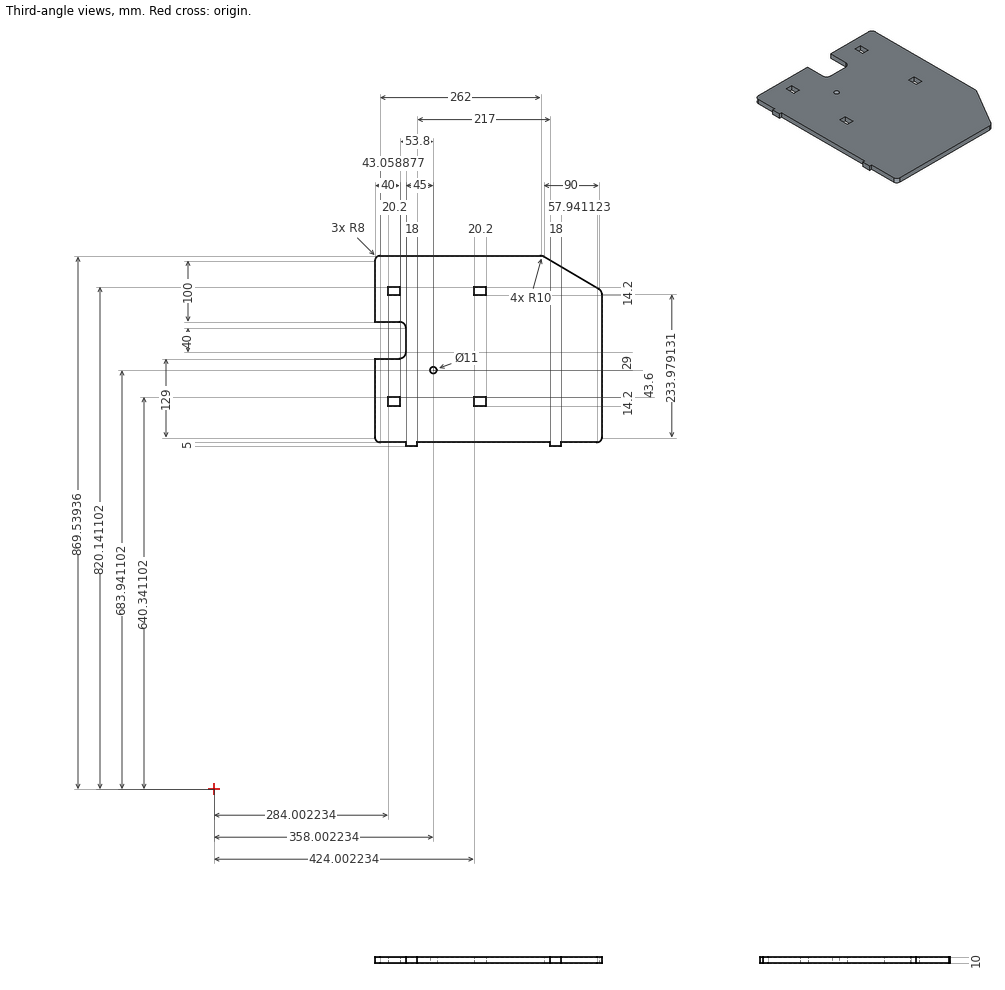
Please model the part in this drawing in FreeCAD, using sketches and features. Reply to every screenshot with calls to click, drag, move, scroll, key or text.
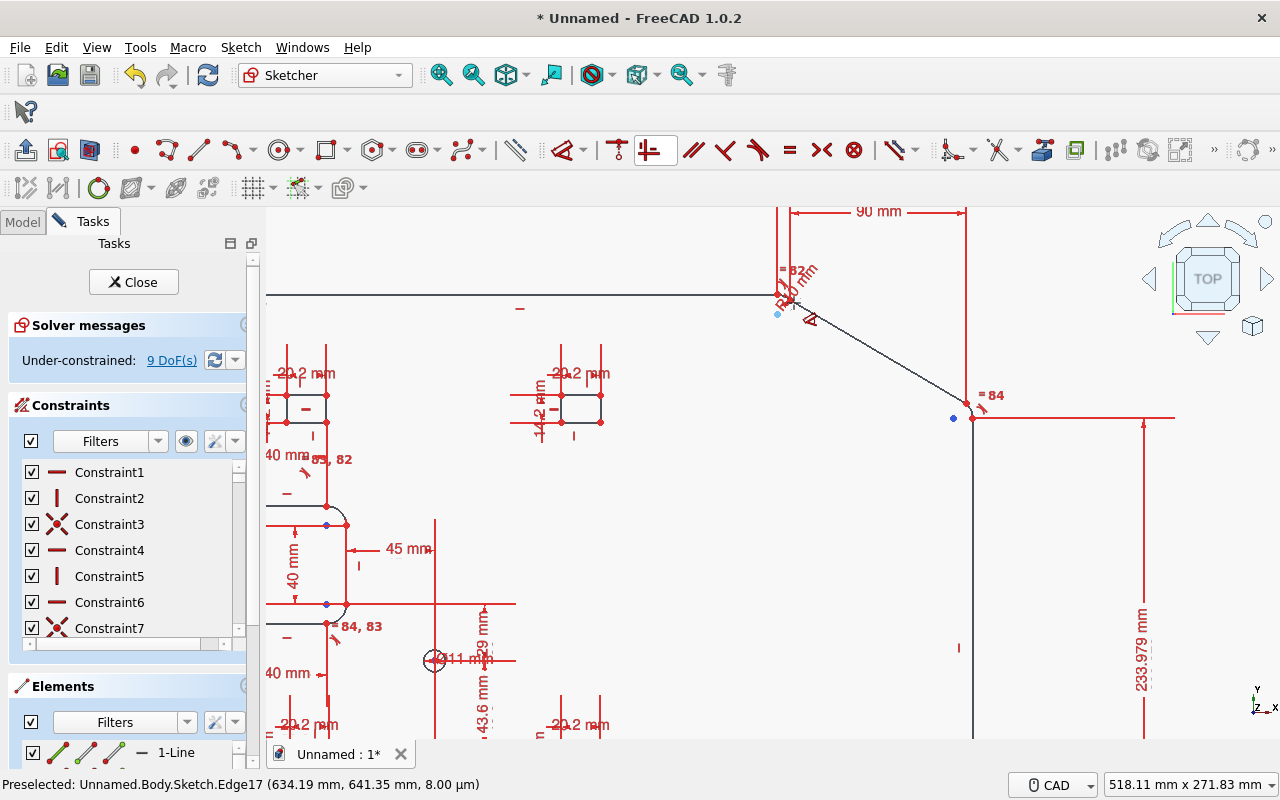
click(790, 300)
click(824, 506)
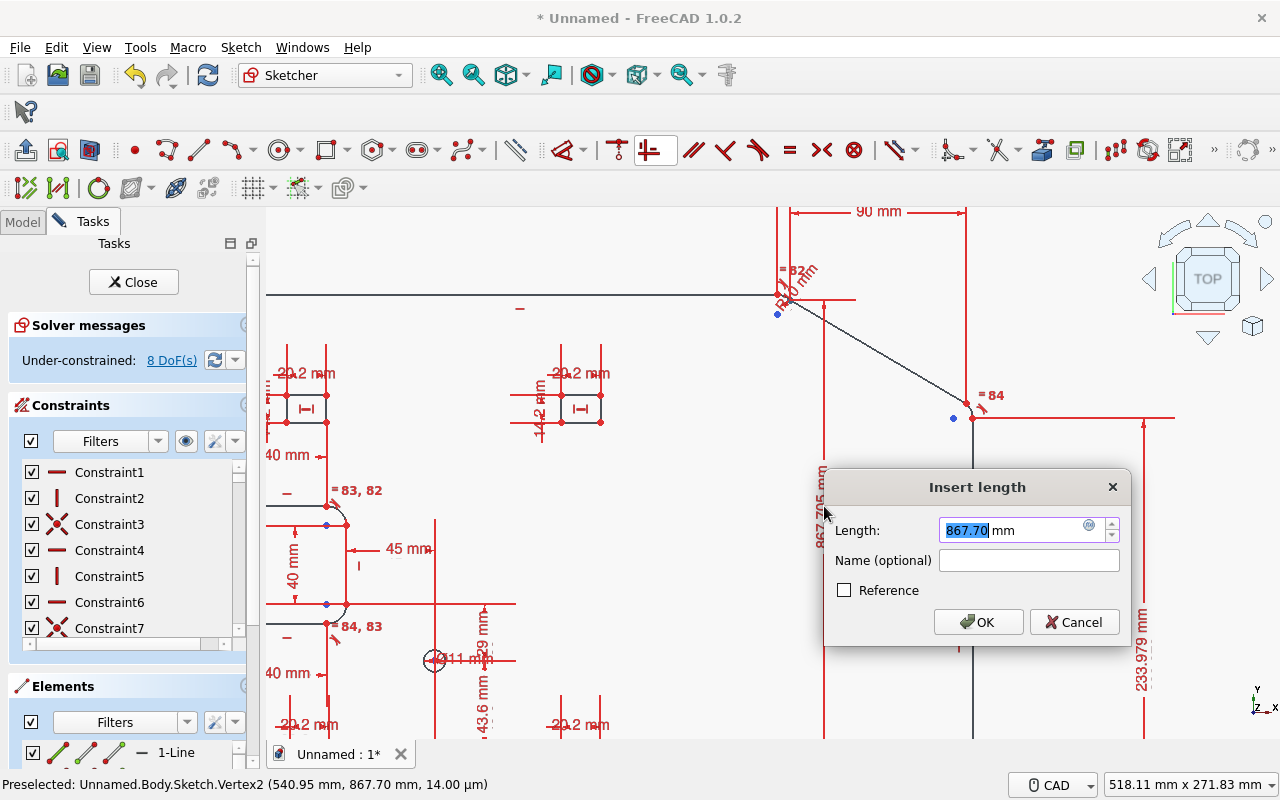
text(869.53936)
key(Return)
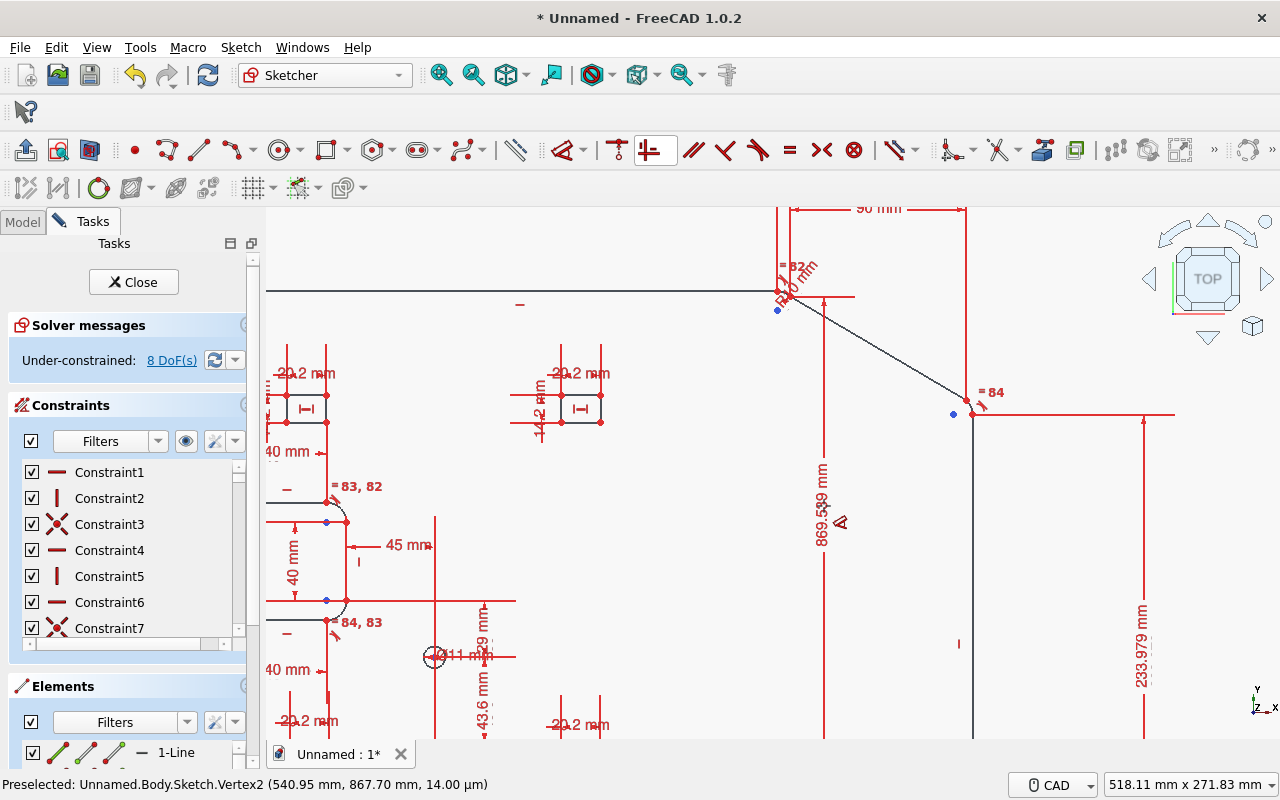
scroll(794, 303, down, 8)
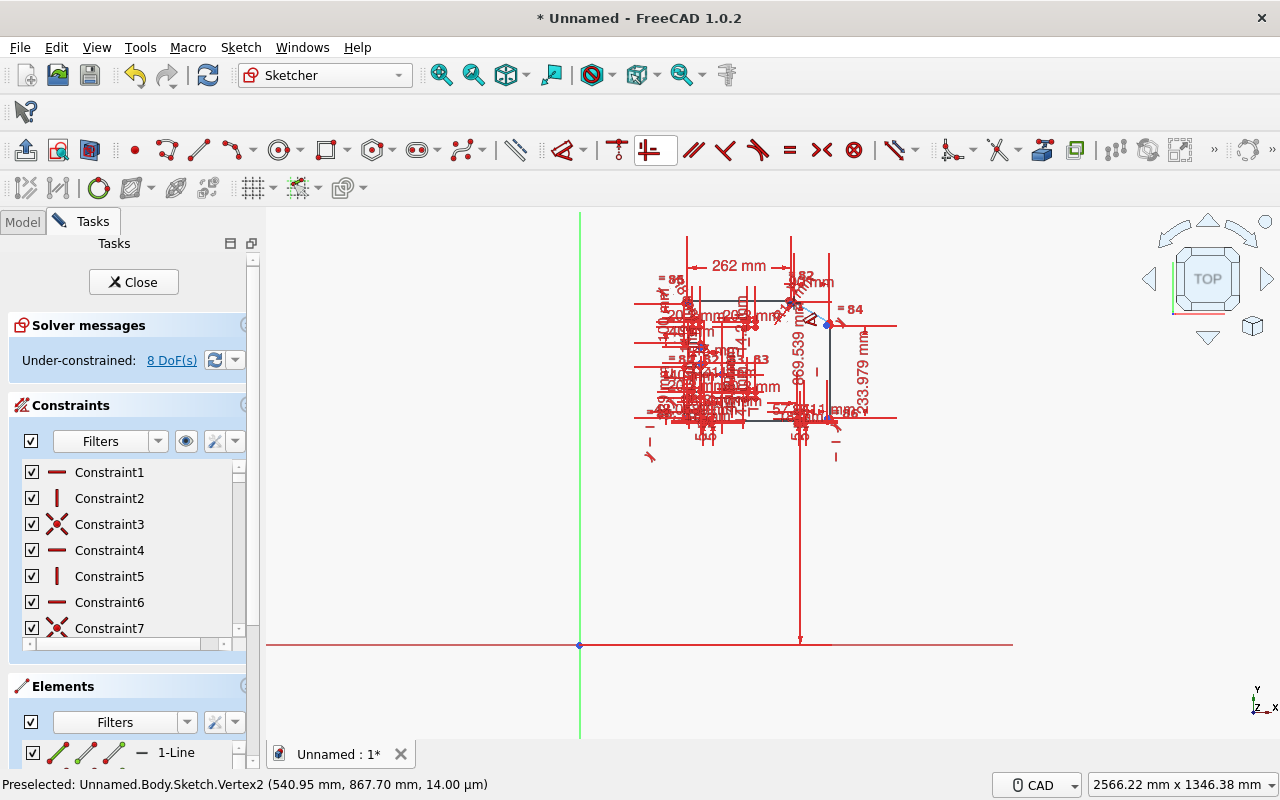
click(722, 375)
click(651, 679)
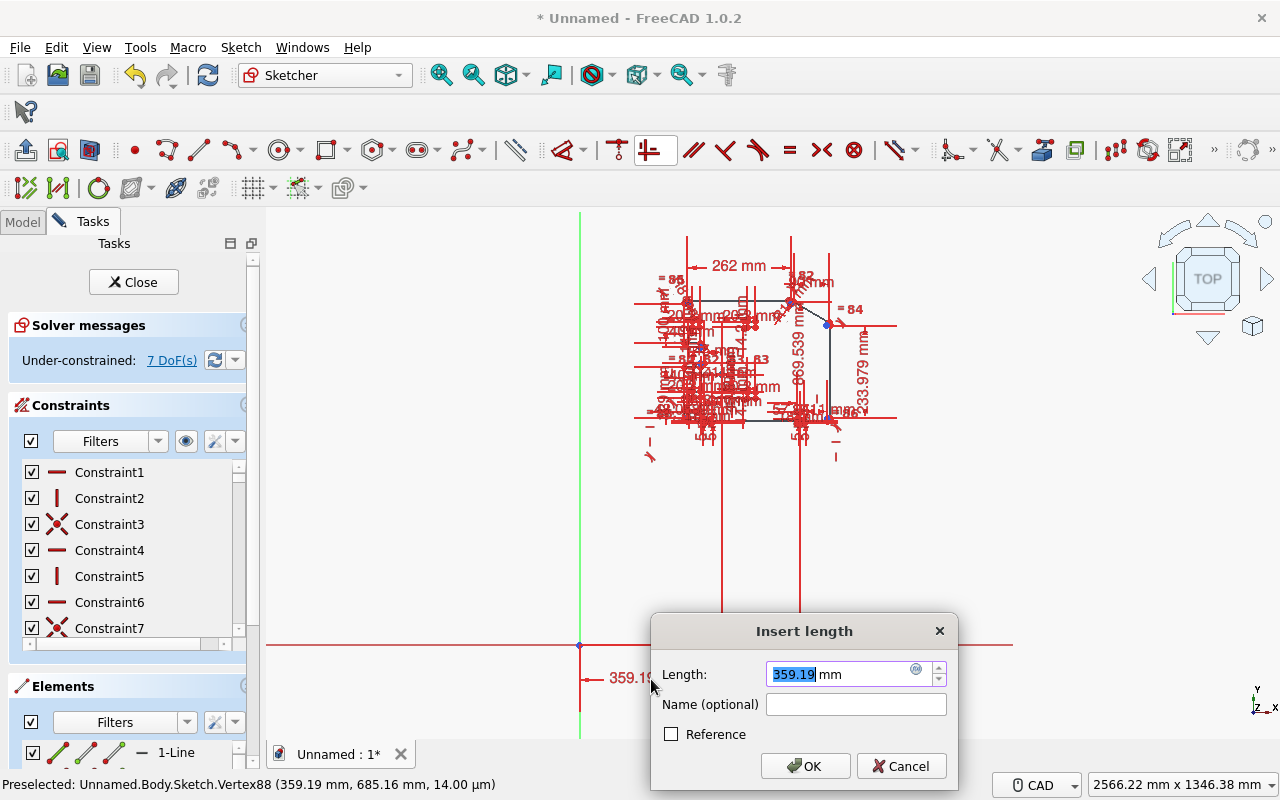
text(358.002234)
key(Return)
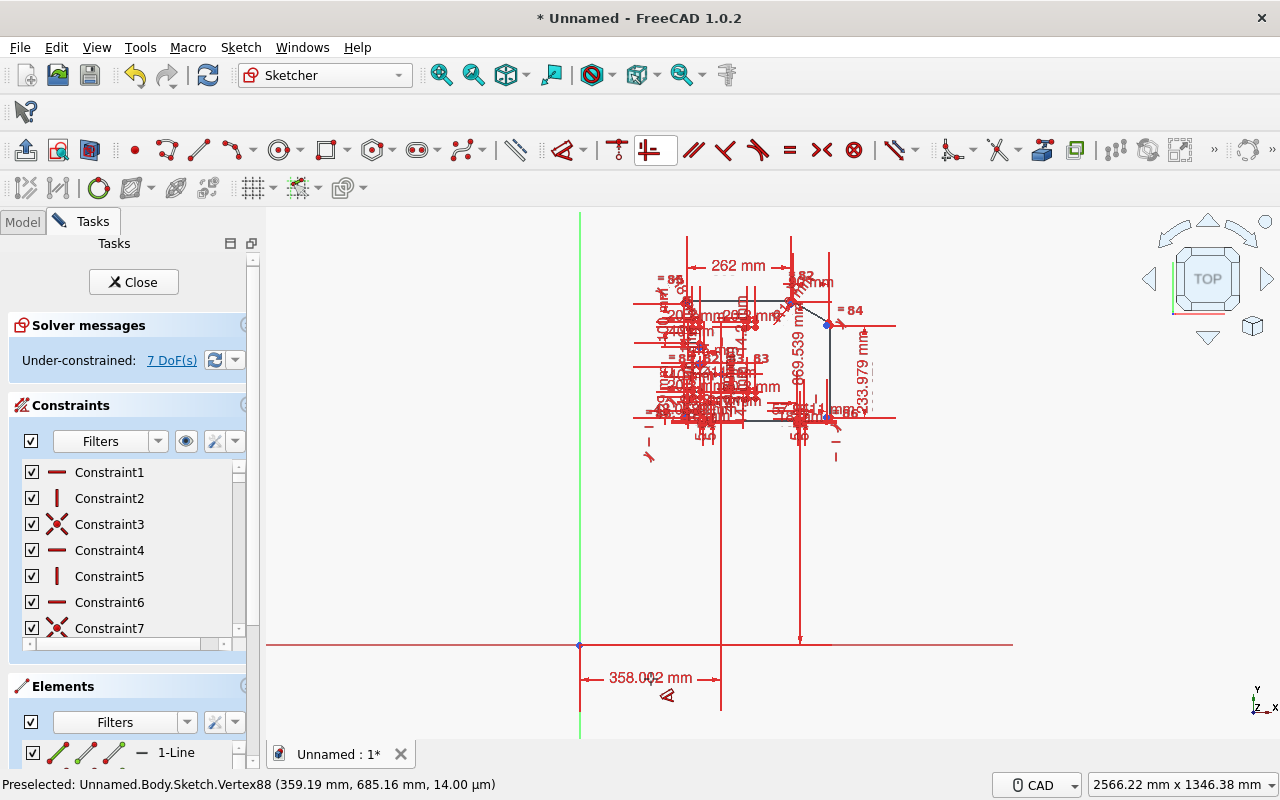
click(721, 374)
click(546, 510)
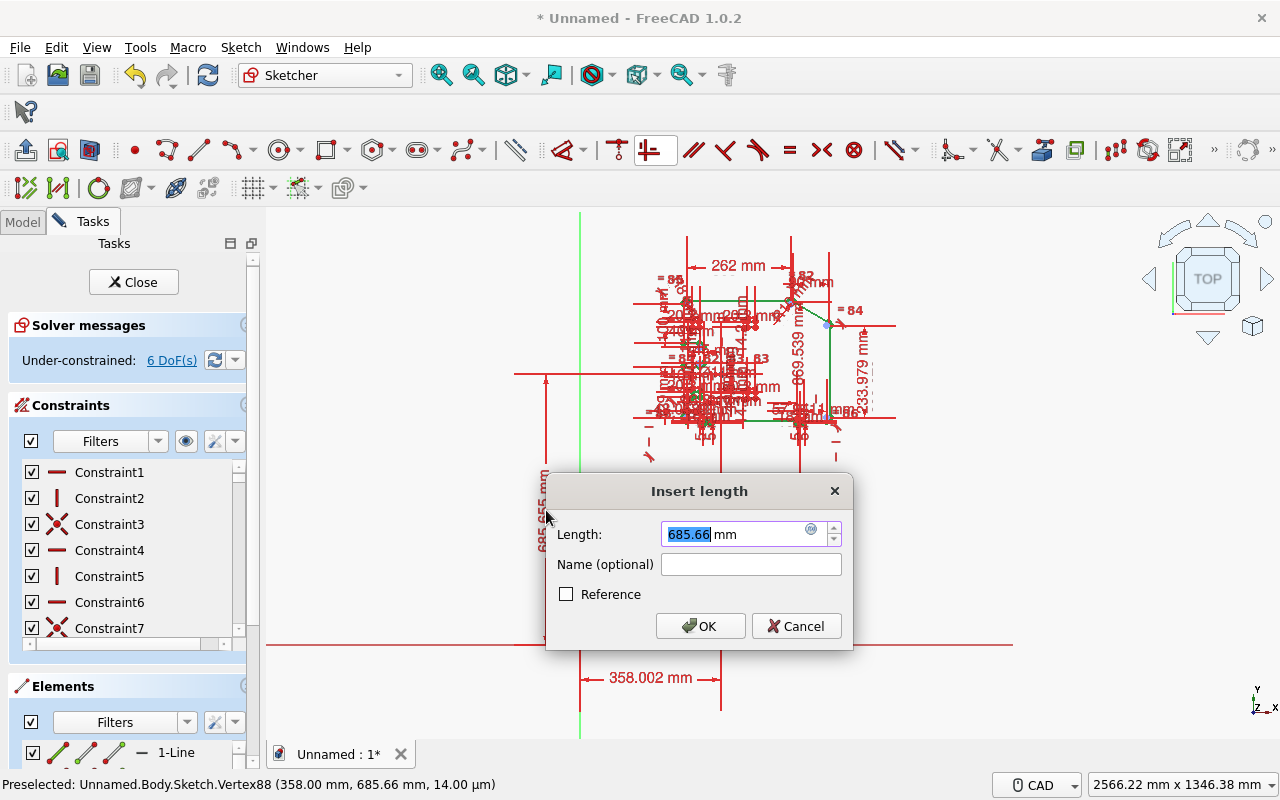
text(683.941102)
key(Return)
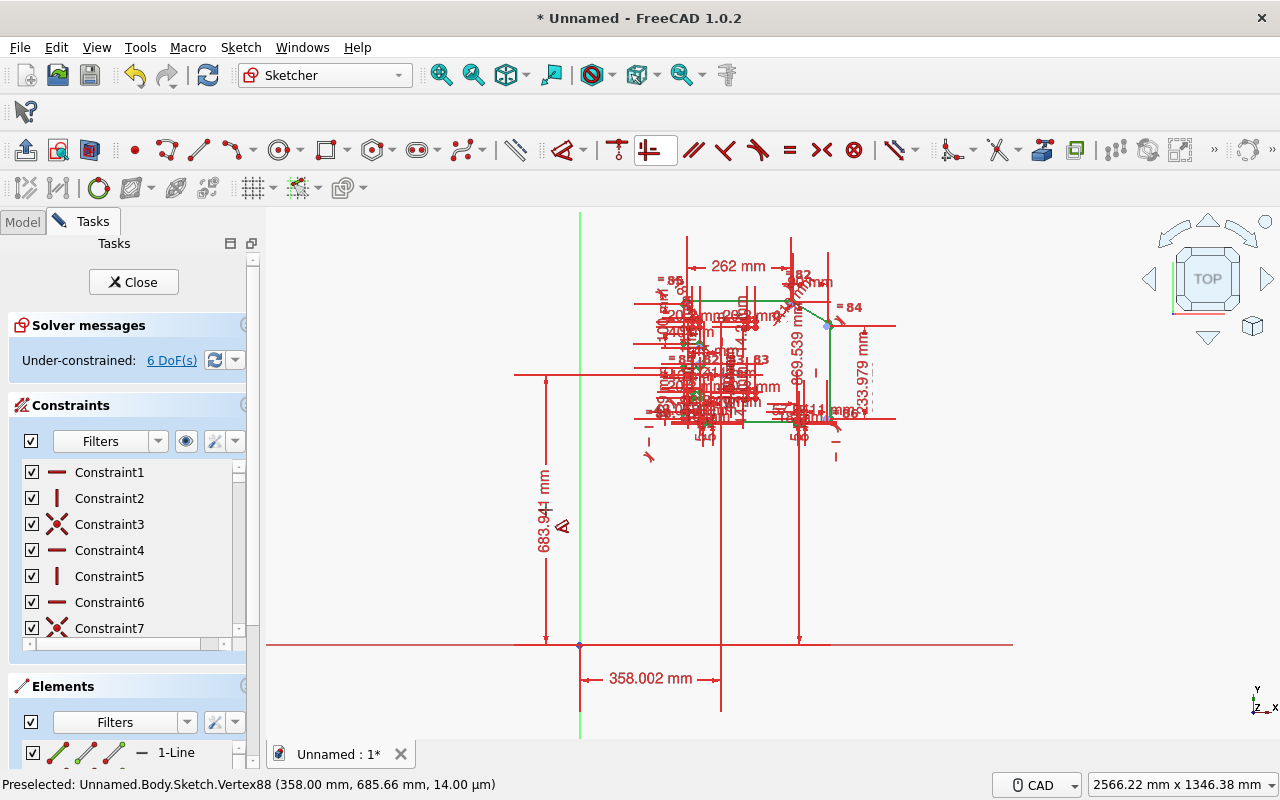
scroll(747, 393, up, 4)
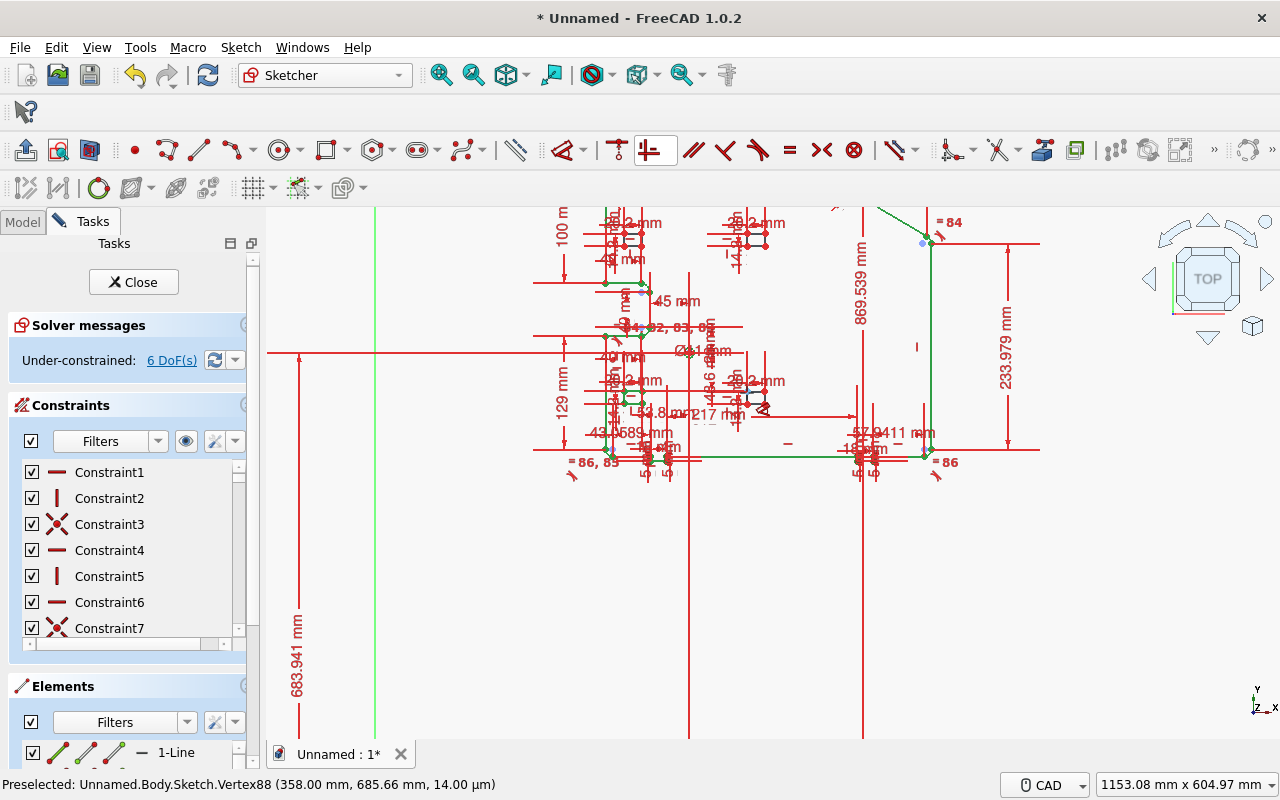
click(747, 392)
click(475, 358)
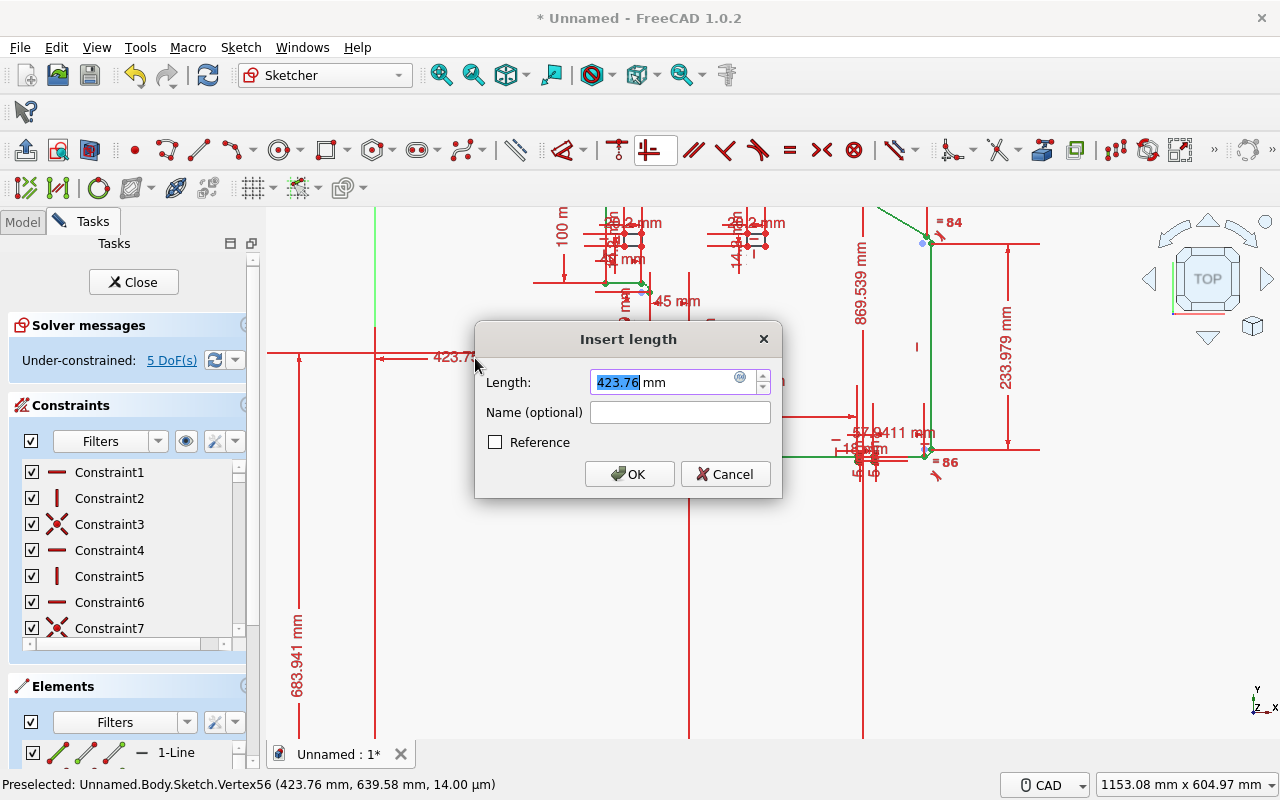
text(424.002234)
key(Return)